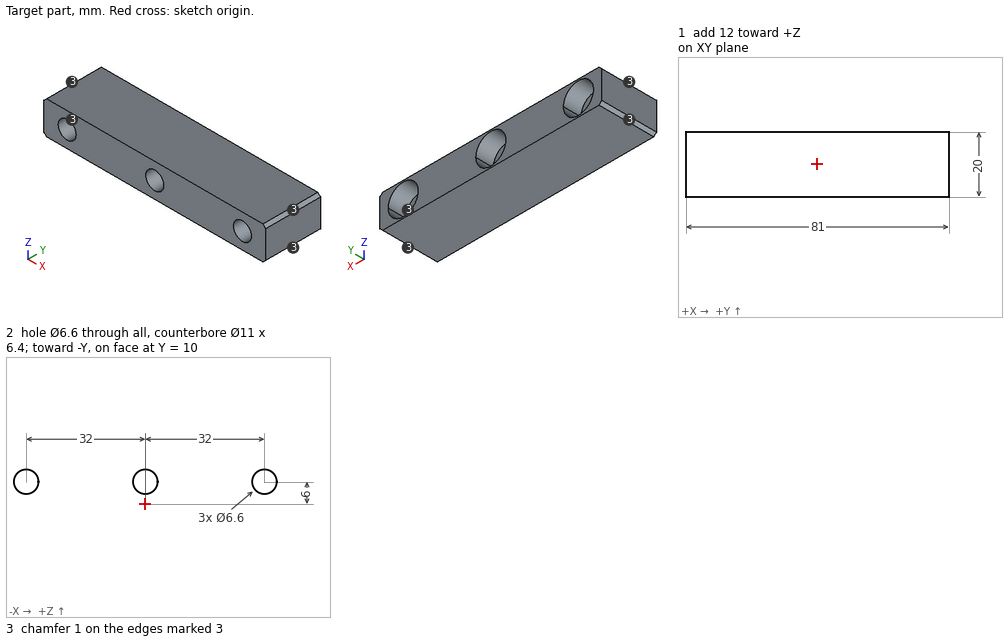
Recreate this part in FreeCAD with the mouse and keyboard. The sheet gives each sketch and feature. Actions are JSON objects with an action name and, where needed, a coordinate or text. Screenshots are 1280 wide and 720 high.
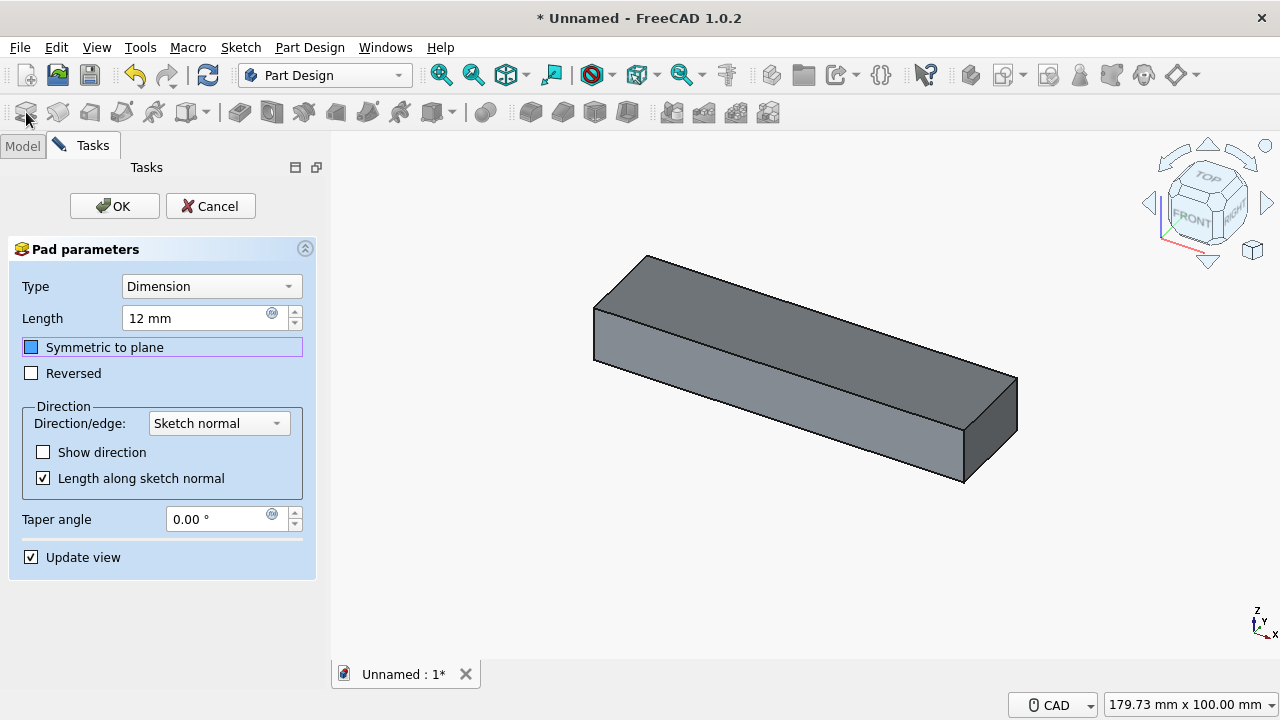
{"action": "left_click", "coordinate": [115, 206]}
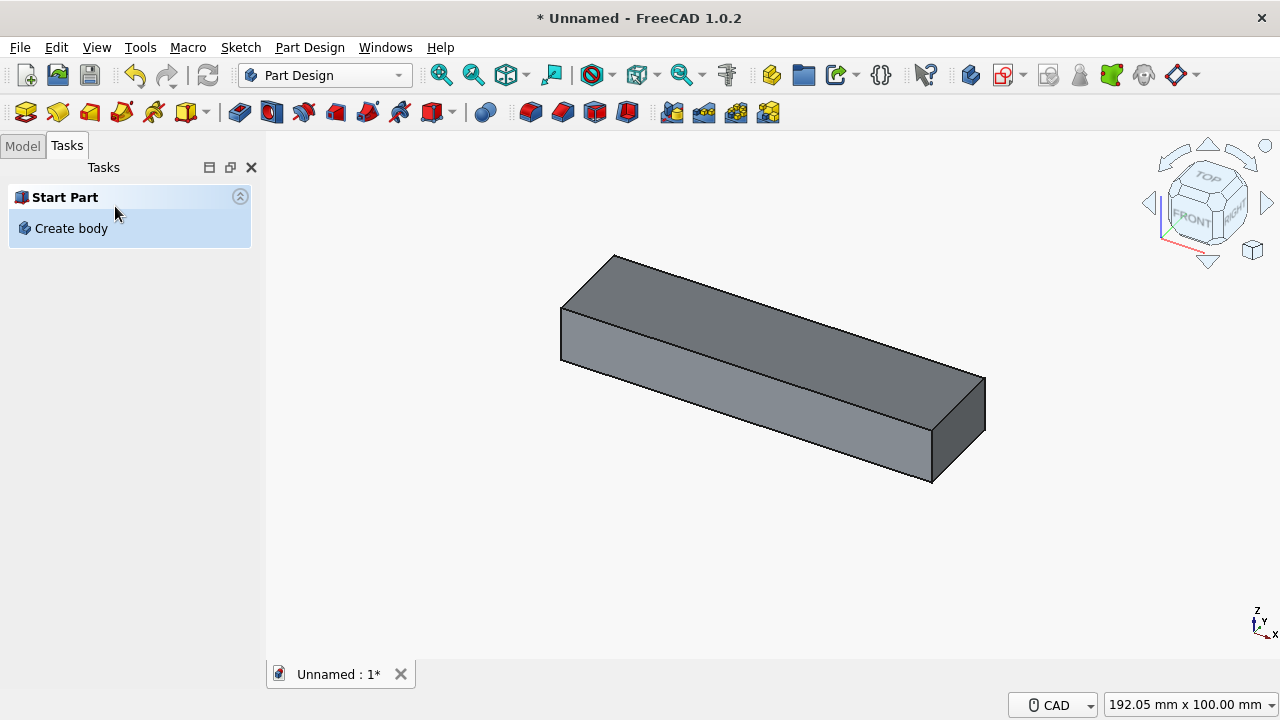
{"action": "left_click", "coordinate": [442, 76]}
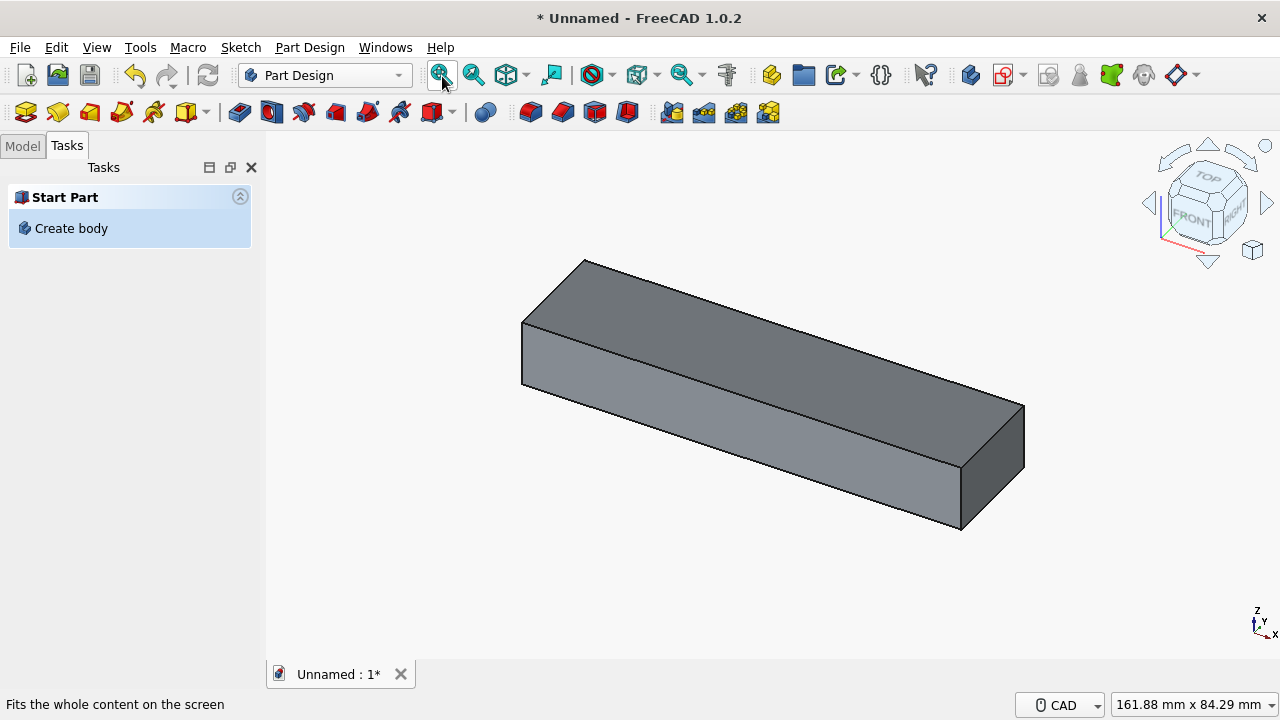
{"action": "key", "text": "4"}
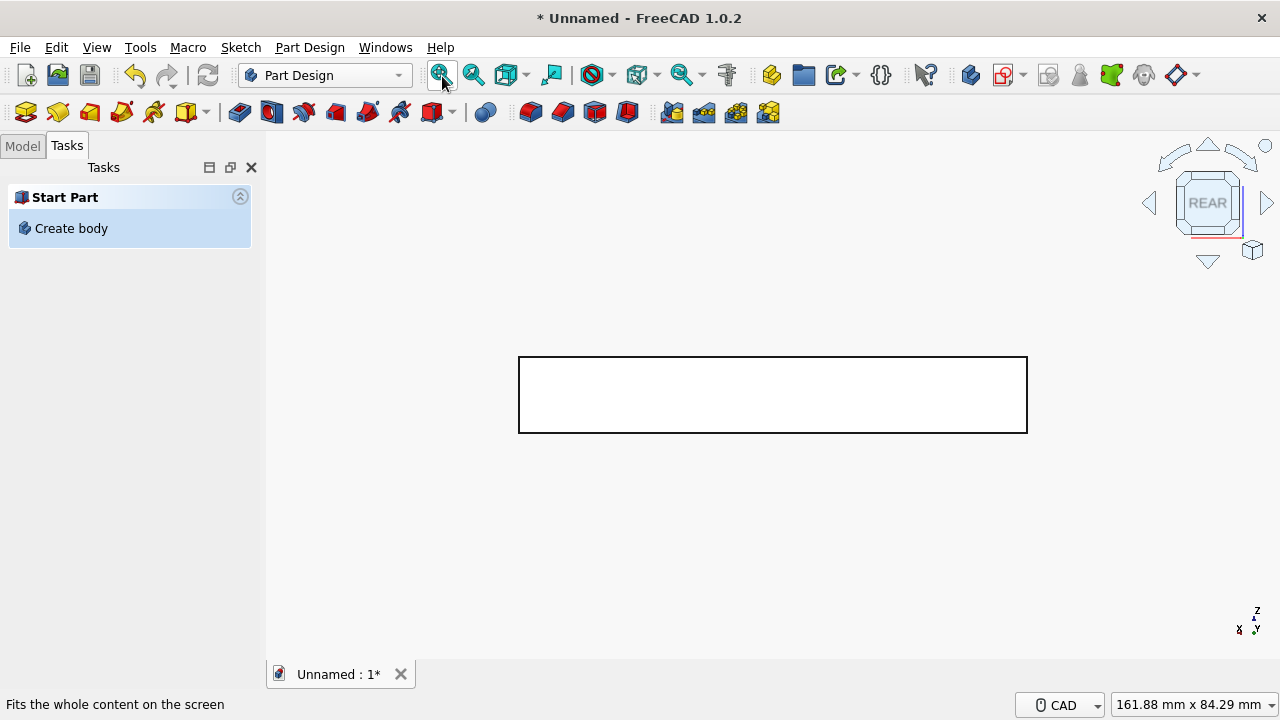
{"action": "left_click", "coordinate": [628, 394]}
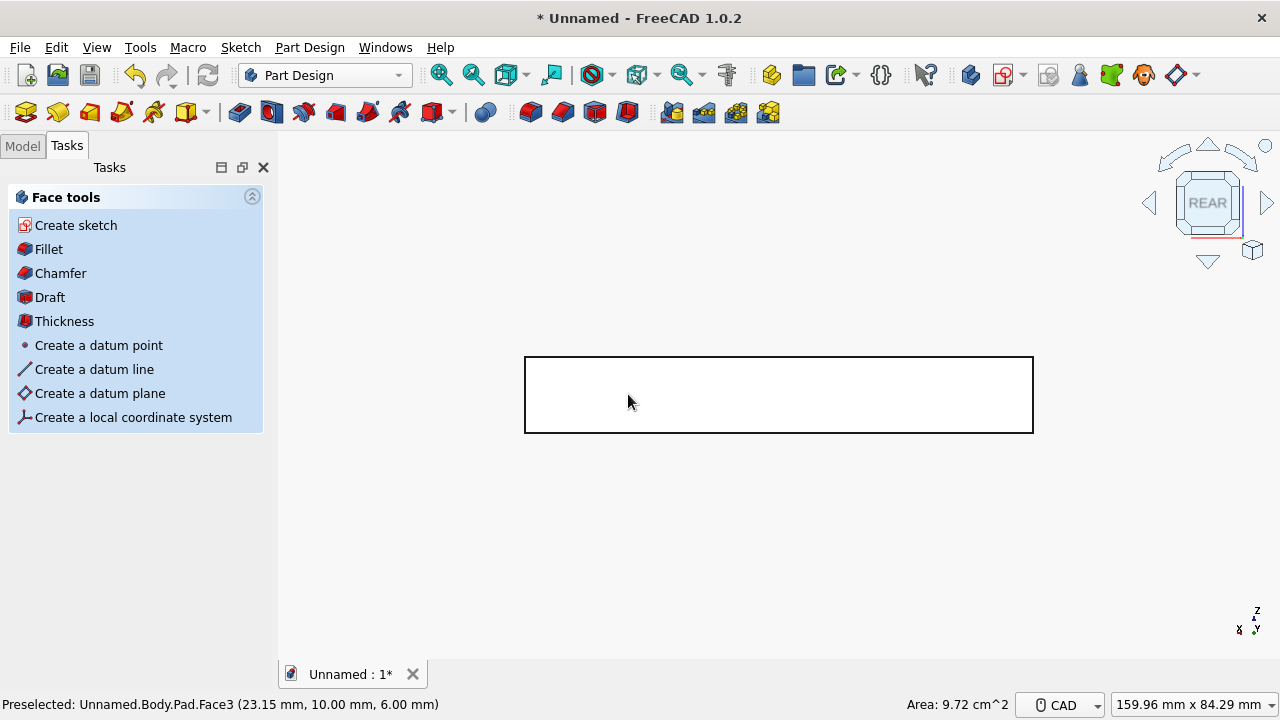
{"action": "left_click", "coordinate": [1004, 76]}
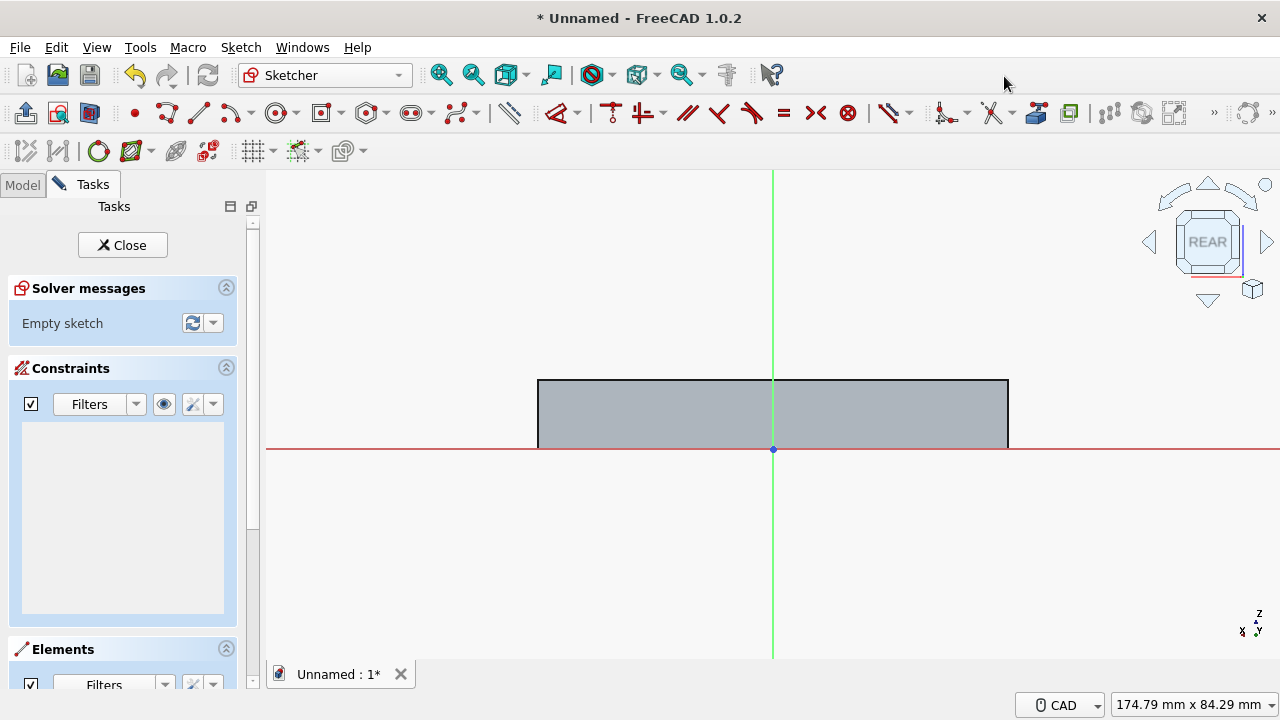
{"action": "scroll", "coordinate": [912, 438], "scroll_direction": "up", "scroll_amount": 2}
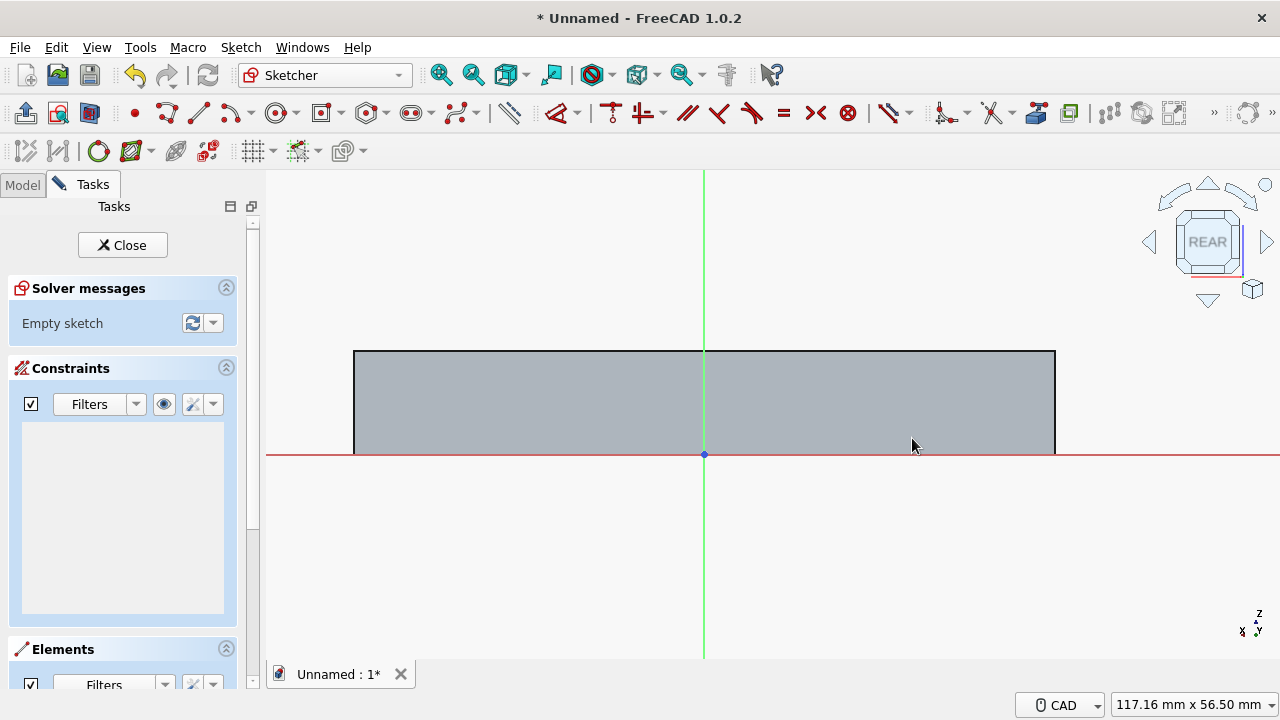
{"action": "left_click", "coordinate": [276, 114]}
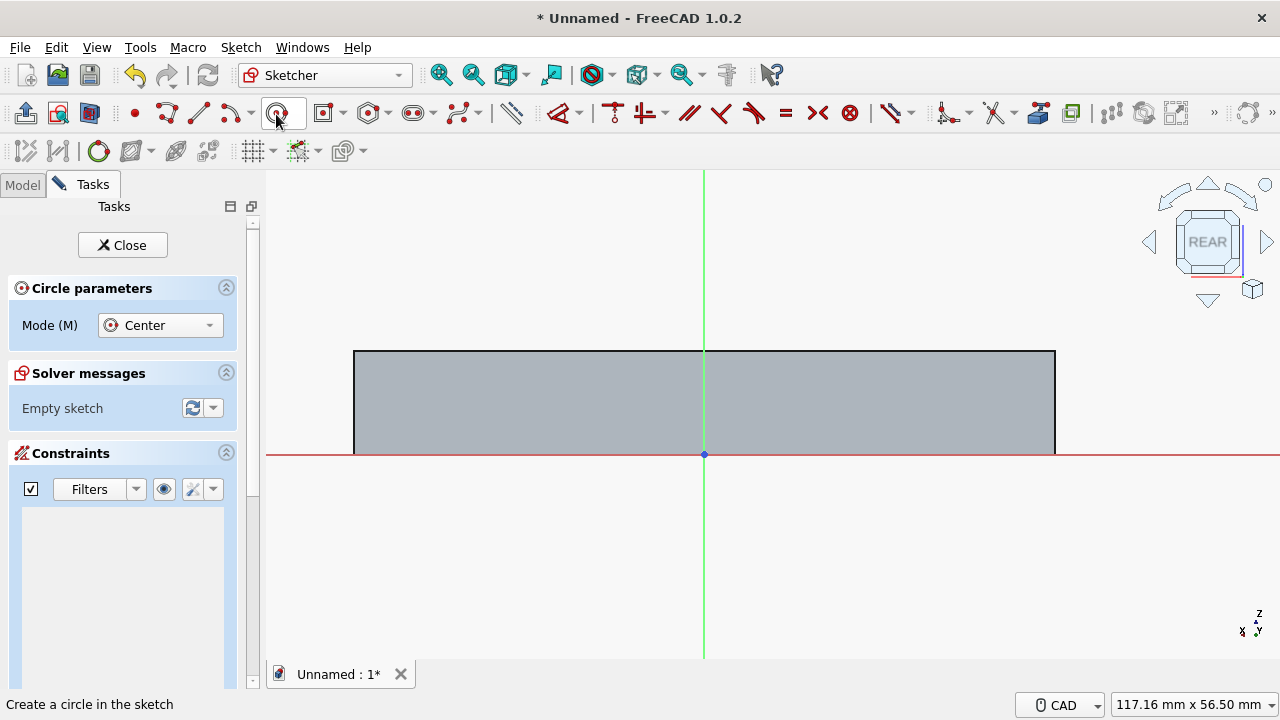
{"action": "left_click", "coordinate": [981, 403]}
{"action": "mouse_move", "coordinate": [1001, 382]}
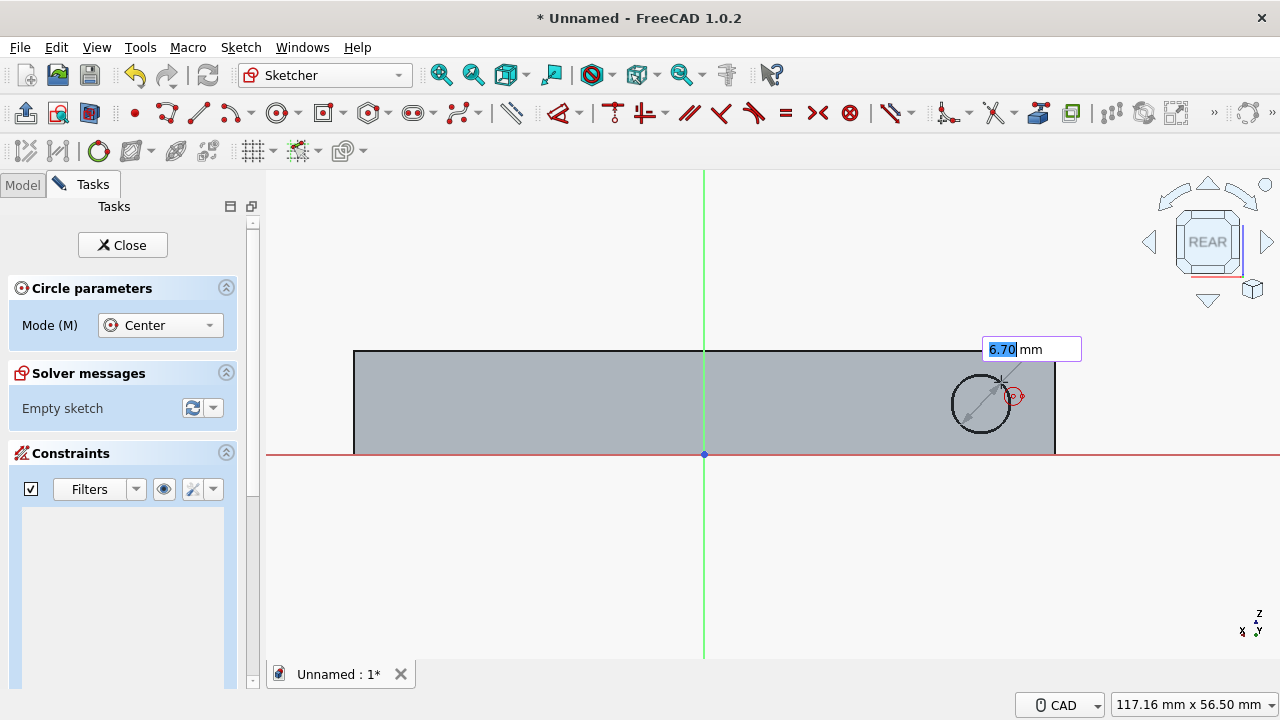
{"action": "type", "text": "6.6"}
{"action": "key", "text": "Return"}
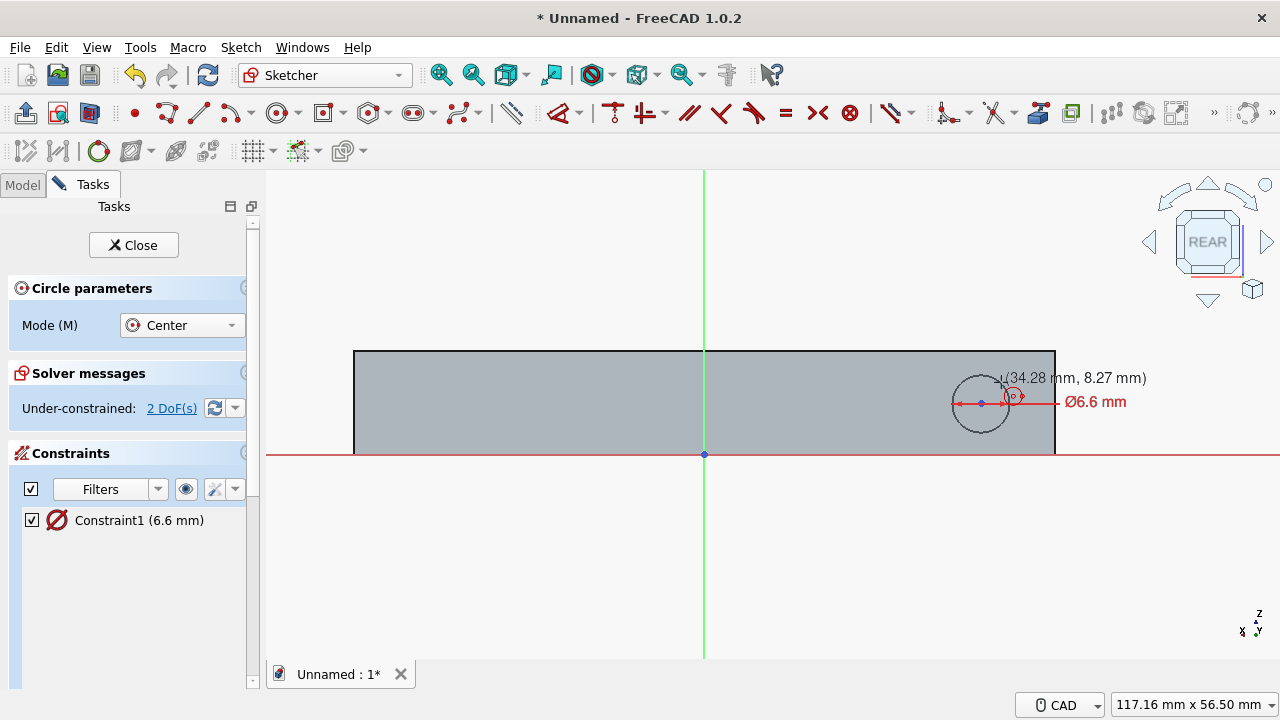
{"action": "left_click", "coordinate": [704, 403]}
{"action": "mouse_move", "coordinate": [725, 382]}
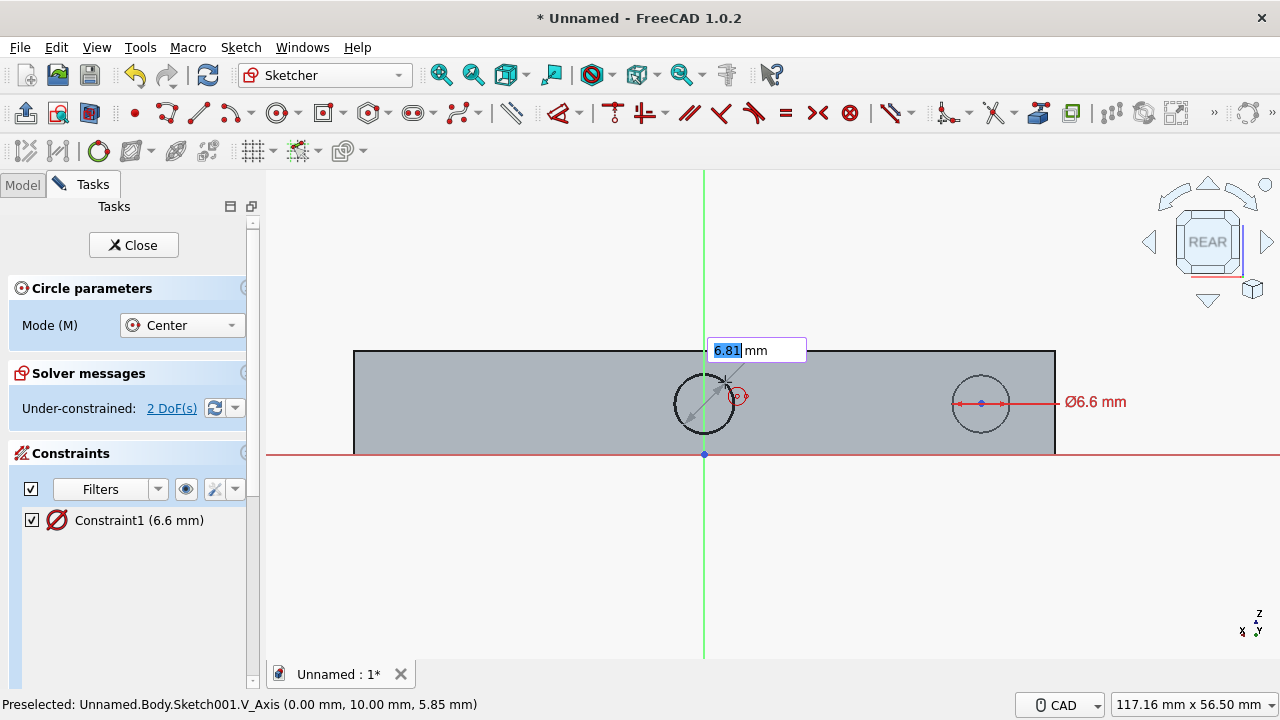
{"action": "type", "text": "6.6"}
{"action": "key", "text": "Return"}